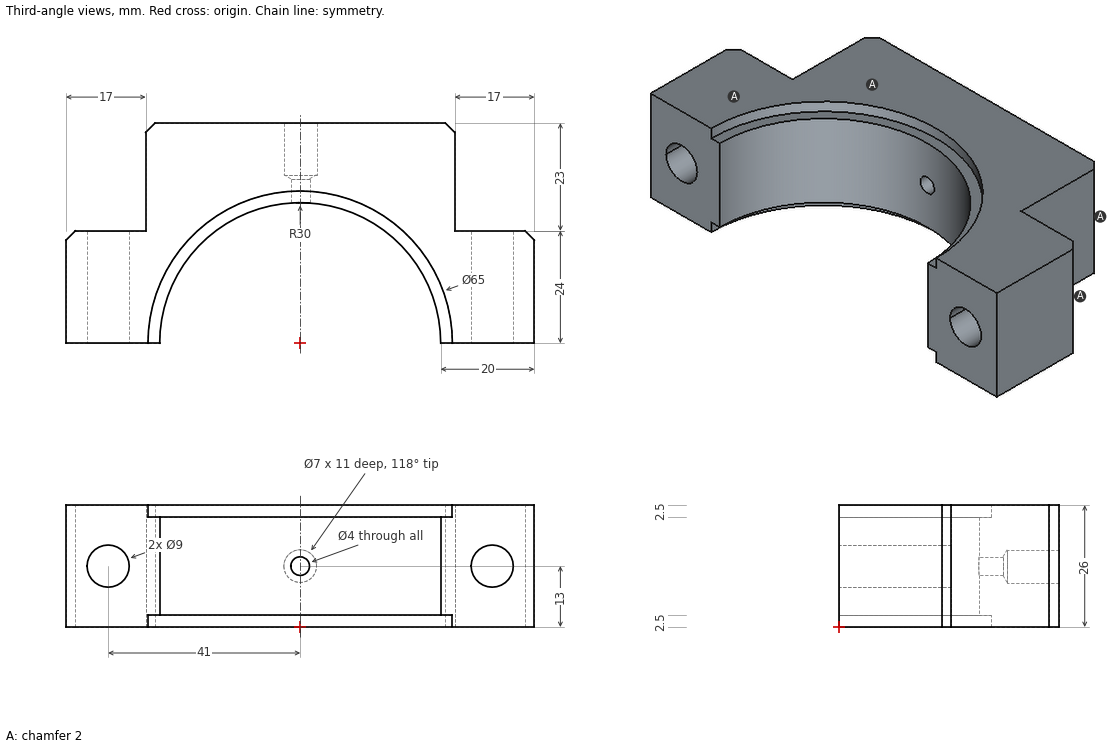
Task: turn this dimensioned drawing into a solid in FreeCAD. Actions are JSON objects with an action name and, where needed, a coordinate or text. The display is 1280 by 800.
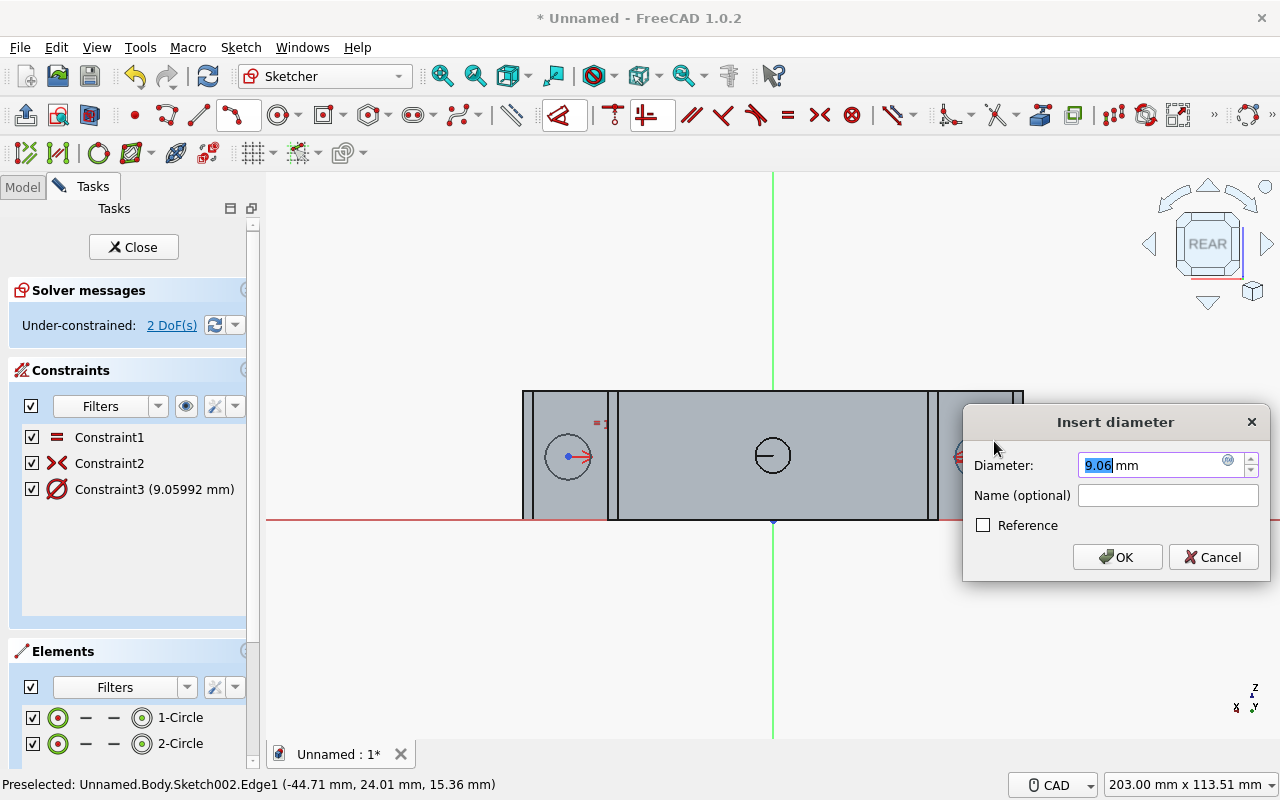
{"action": "type", "text": "9"}
{"action": "key", "text": "Return"}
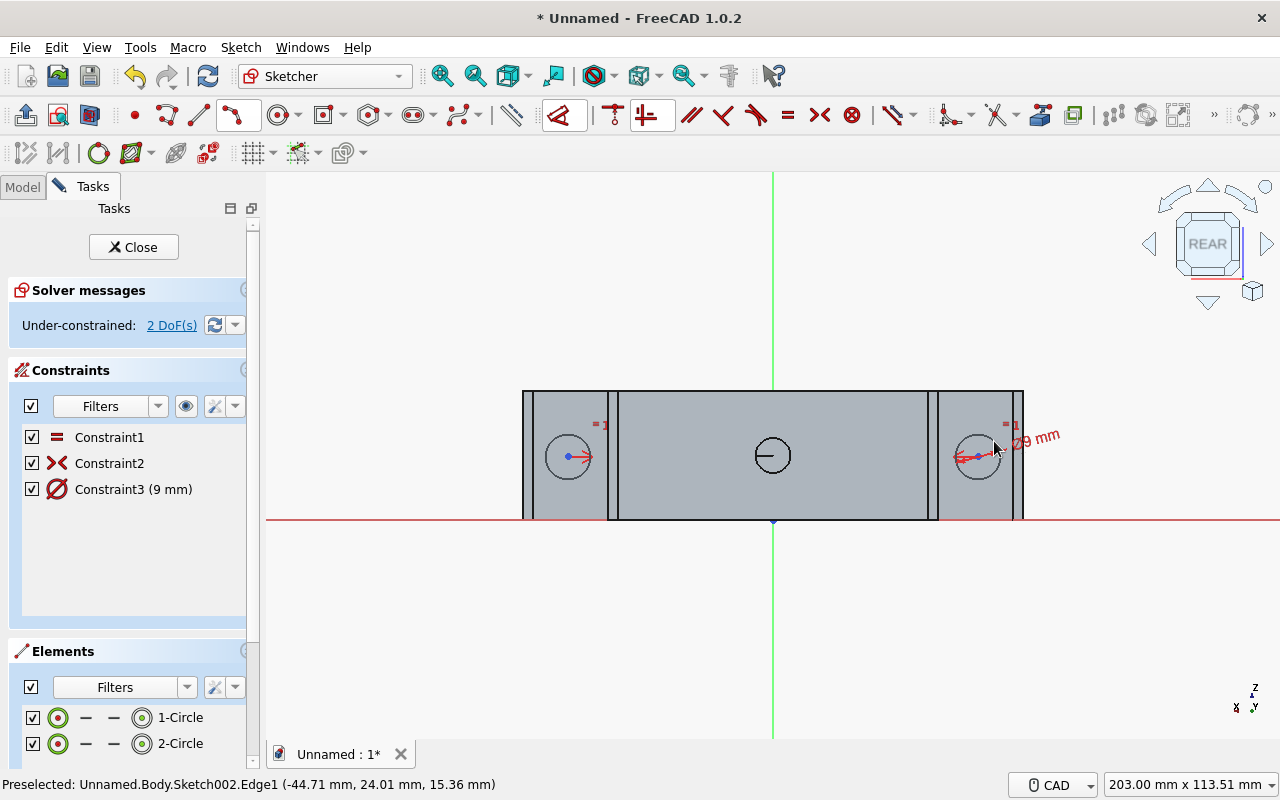
{"action": "left_click", "coordinate": [978, 457]}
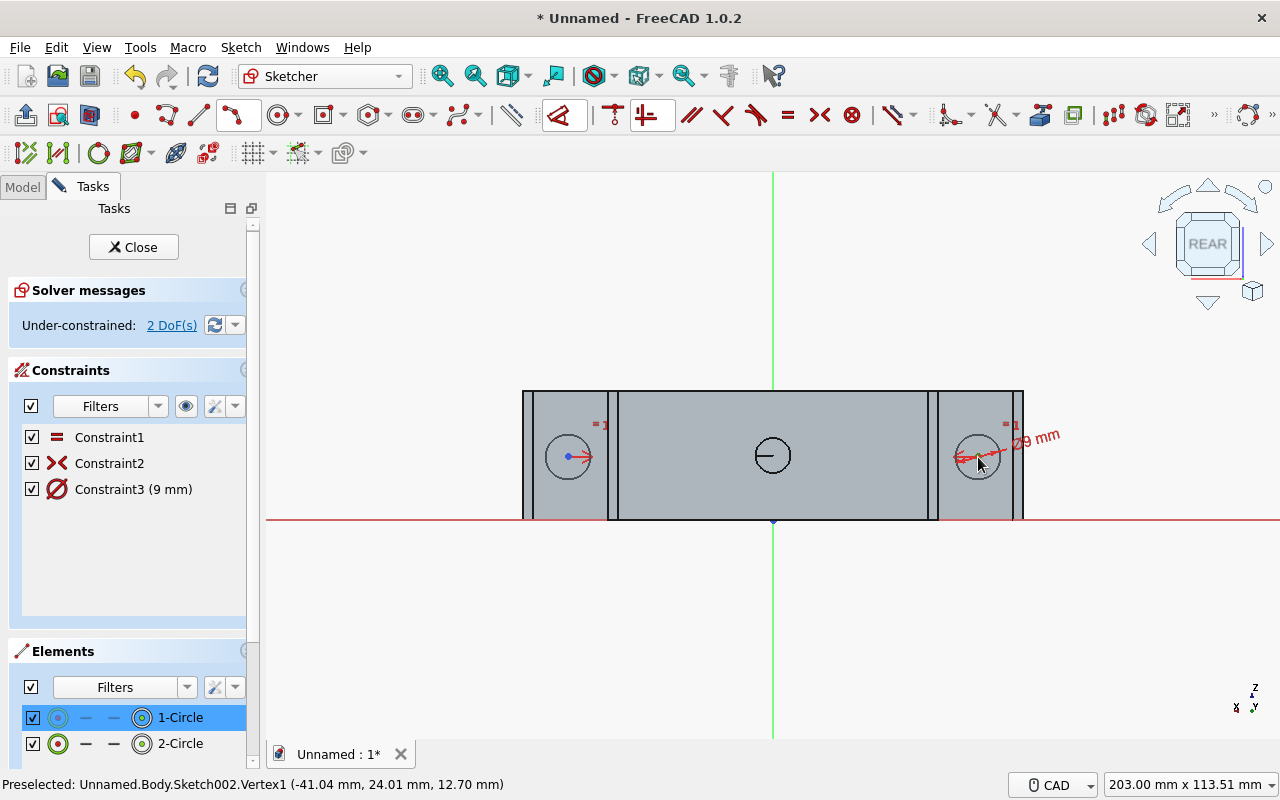
{"action": "key", "text": "l"}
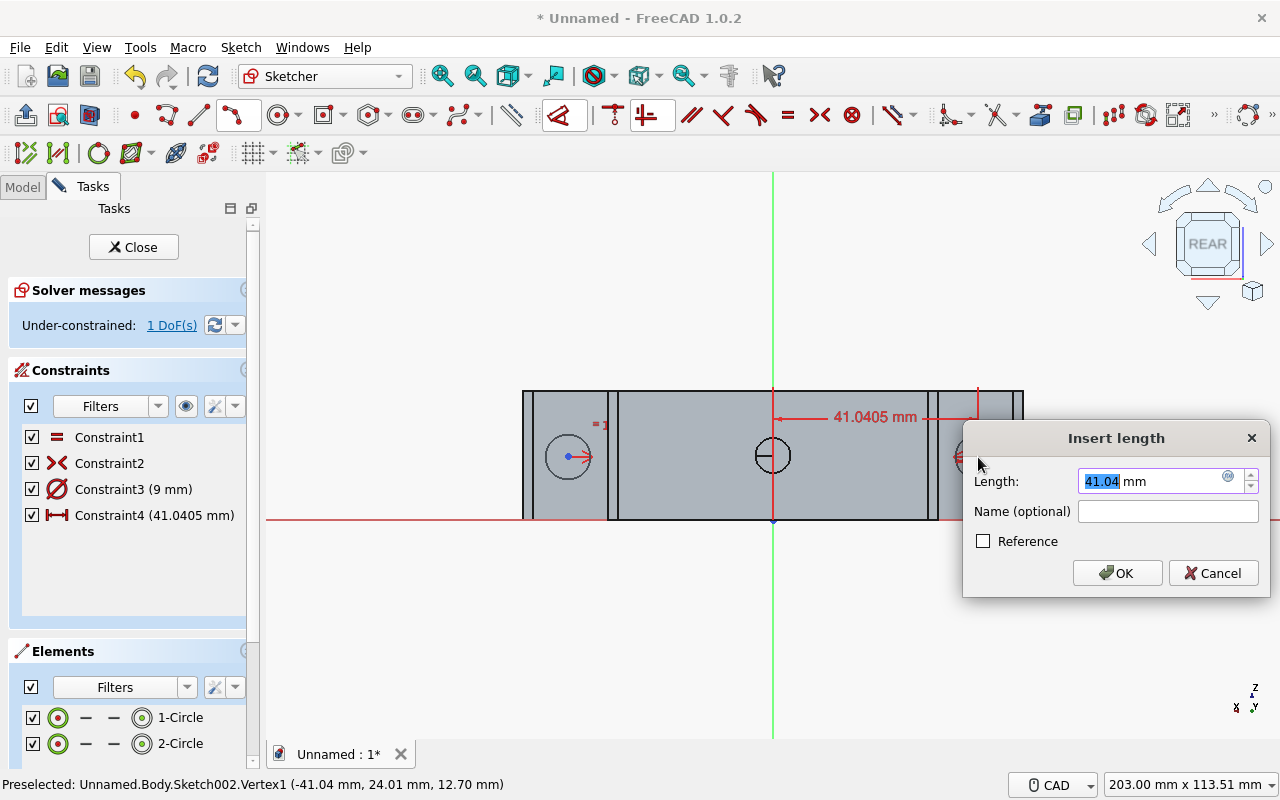
{"action": "type", "text": "41"}
{"action": "key", "text": "Return"}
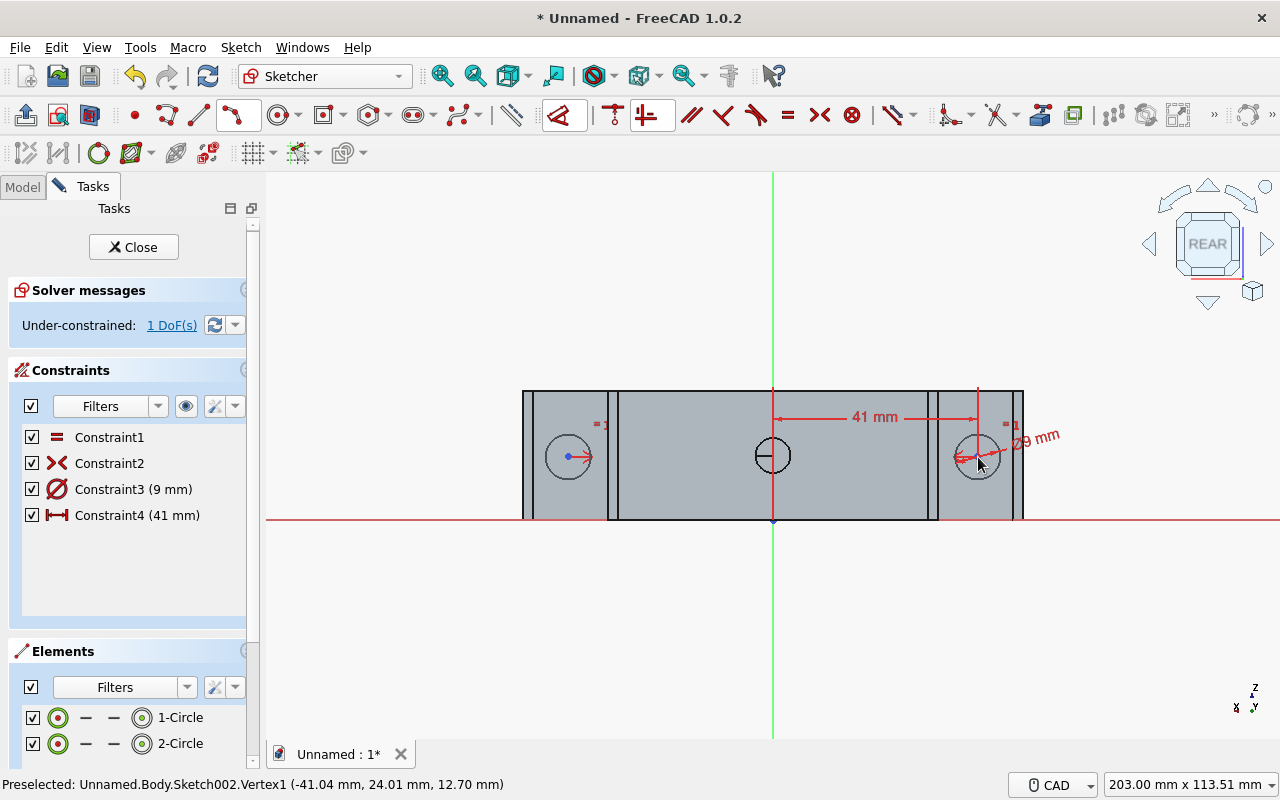
{"action": "left_click", "coordinate": [978, 457]}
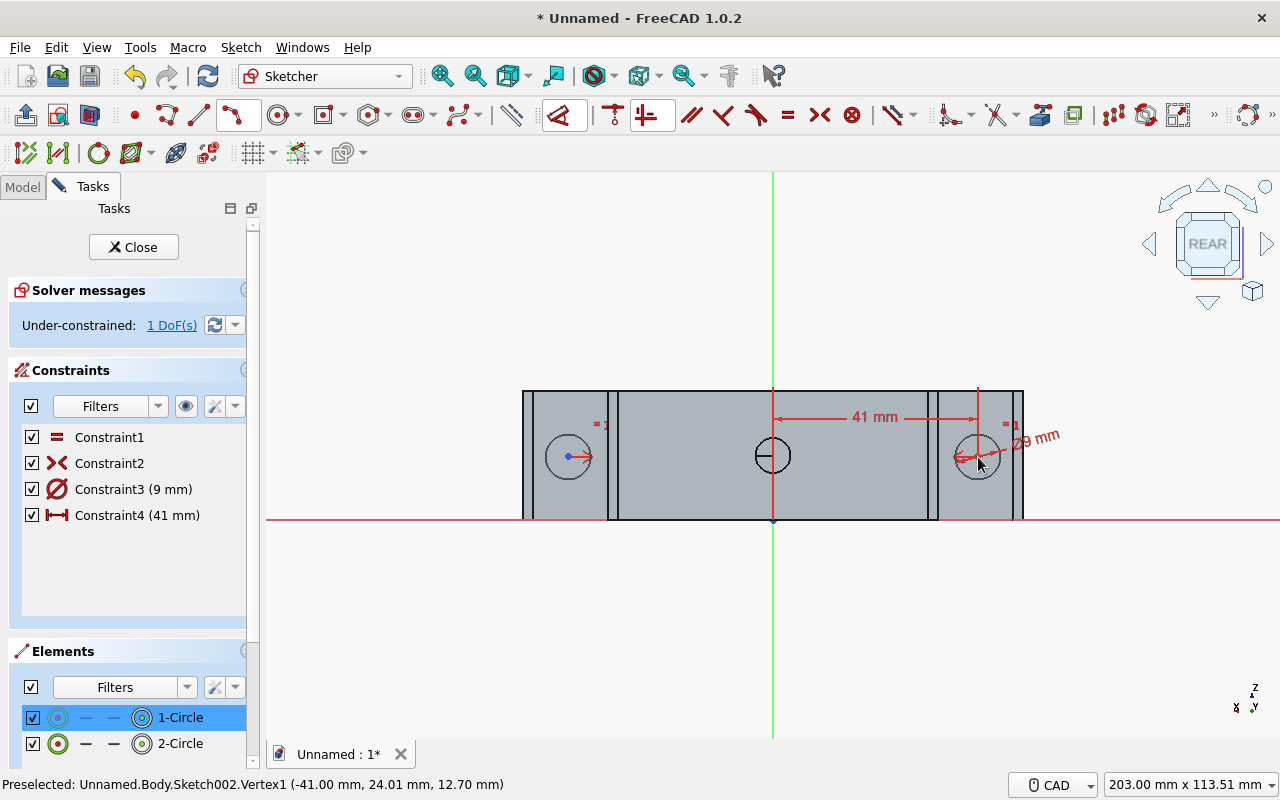
{"action": "key", "text": "i"}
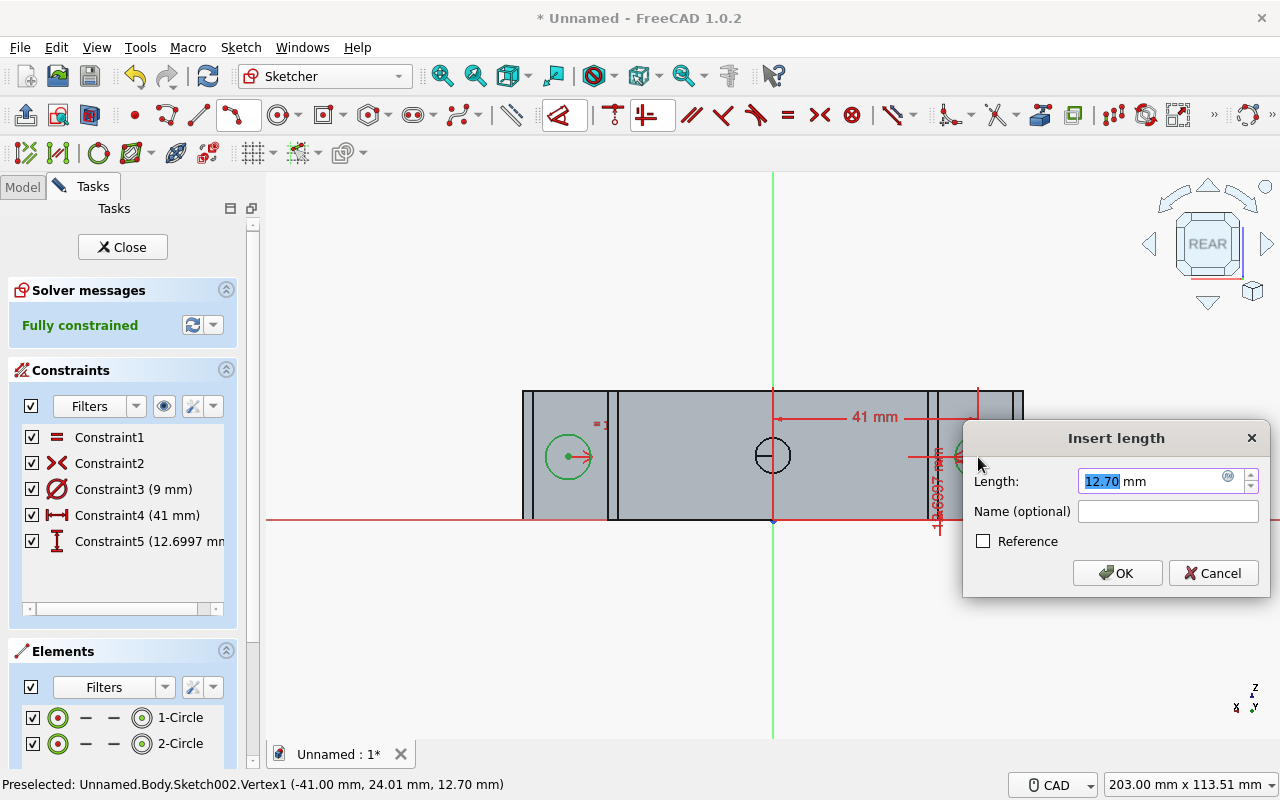
{"action": "type", "text": "13"}
{"action": "key", "text": "Return"}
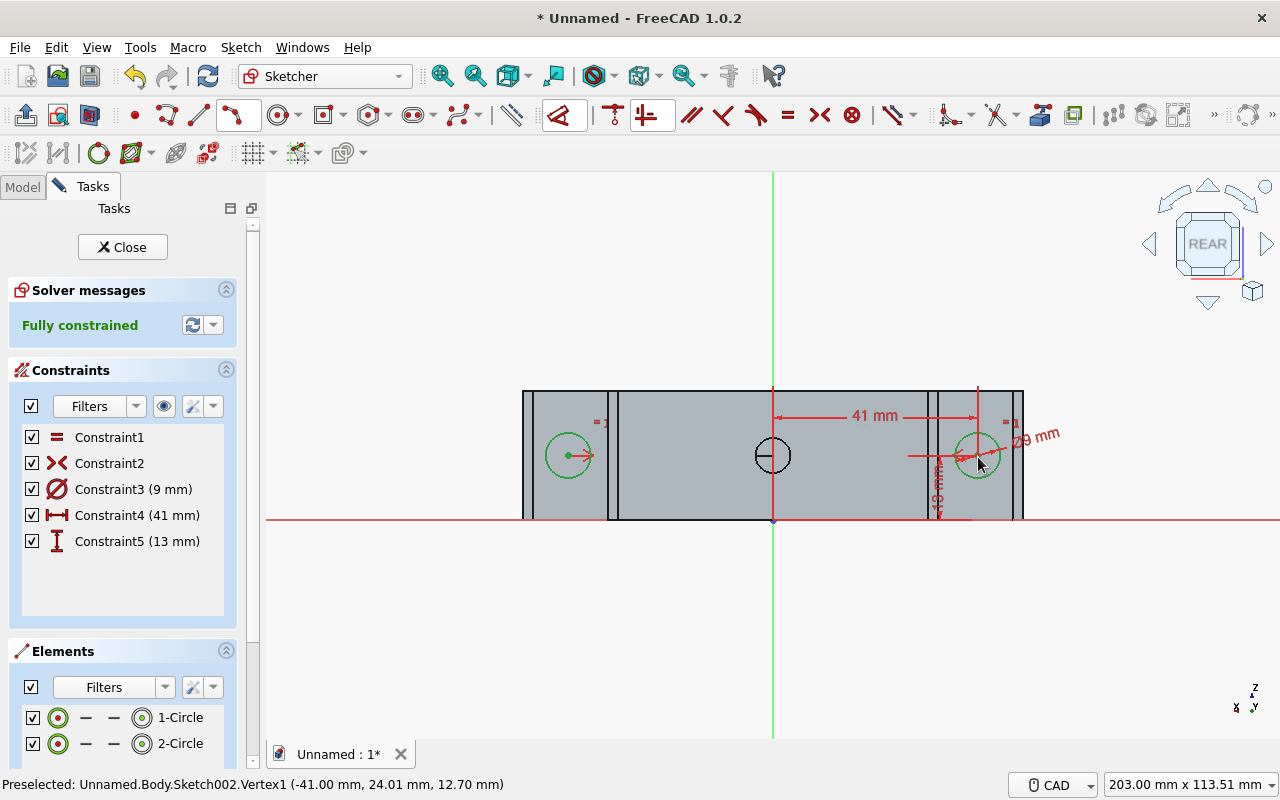
{"action": "left_click", "coordinate": [123, 247]}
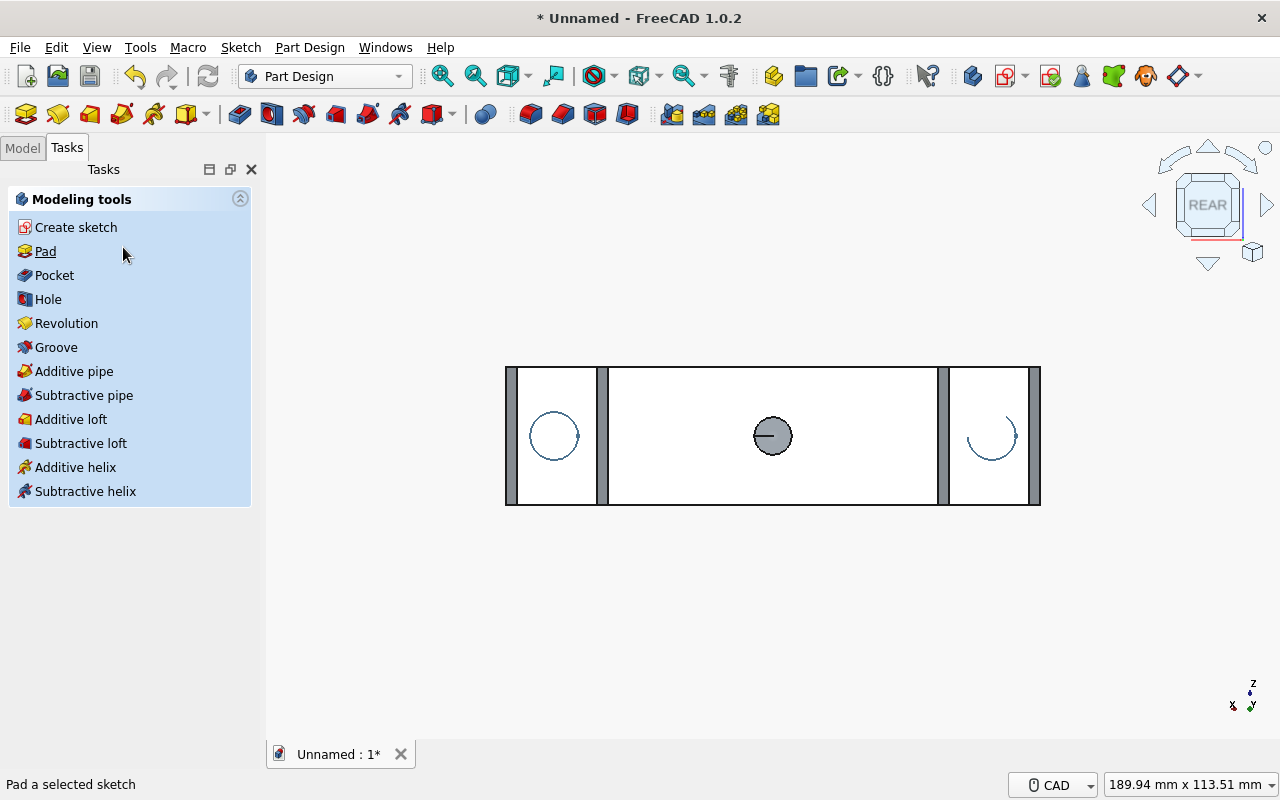
{"action": "left_click", "coordinate": [240, 114]}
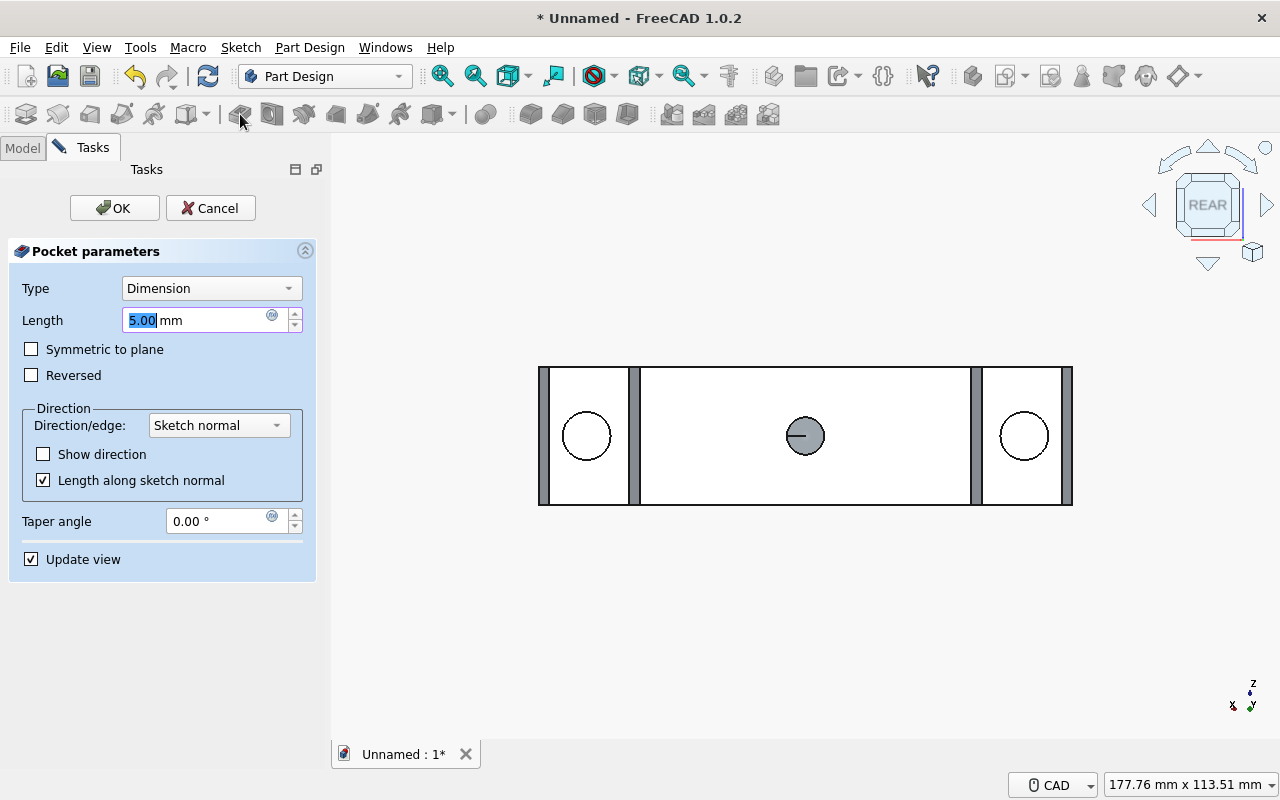
{"action": "left_click", "coordinate": [212, 288]}